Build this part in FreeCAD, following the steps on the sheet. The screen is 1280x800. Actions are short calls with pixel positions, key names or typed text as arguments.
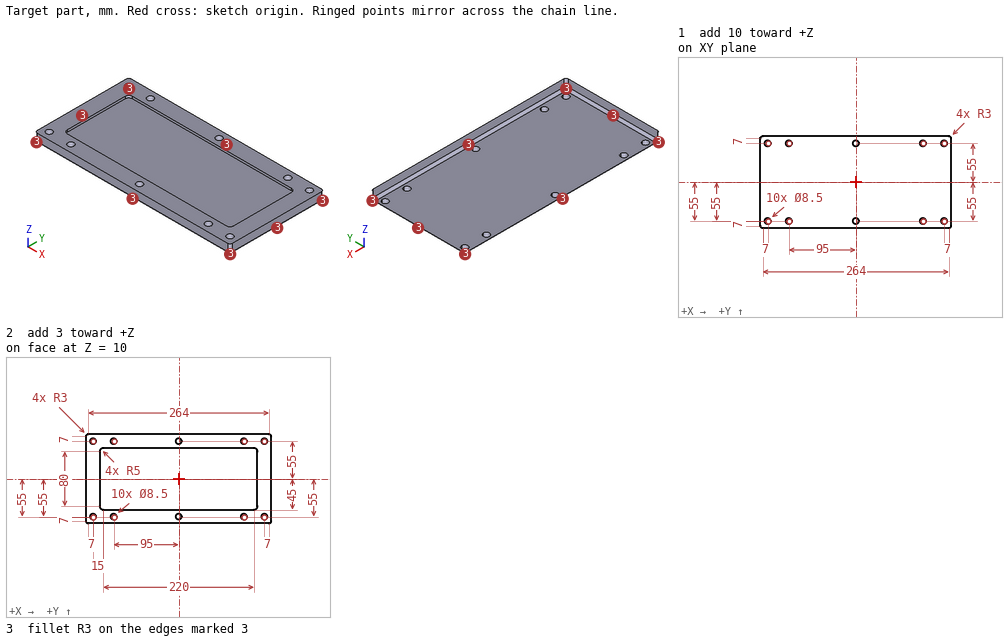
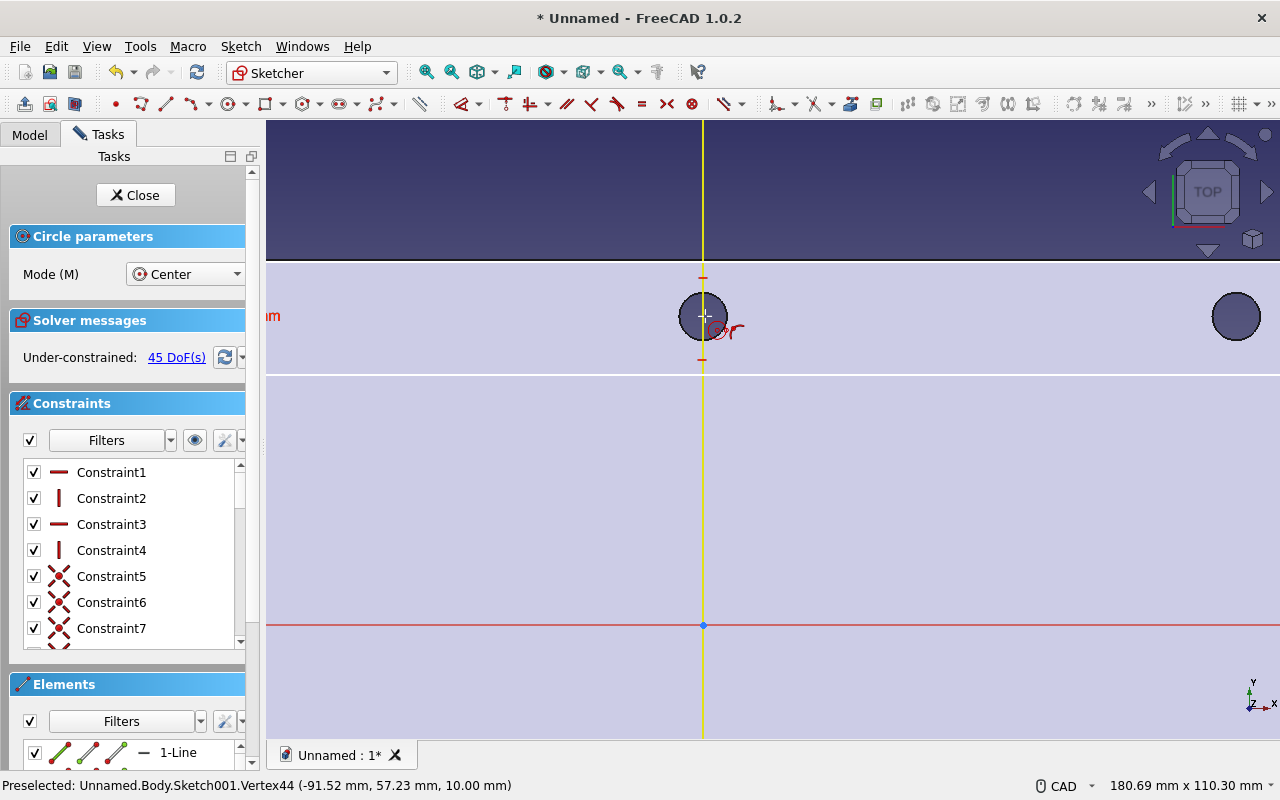
click(703, 317)
move(720, 300)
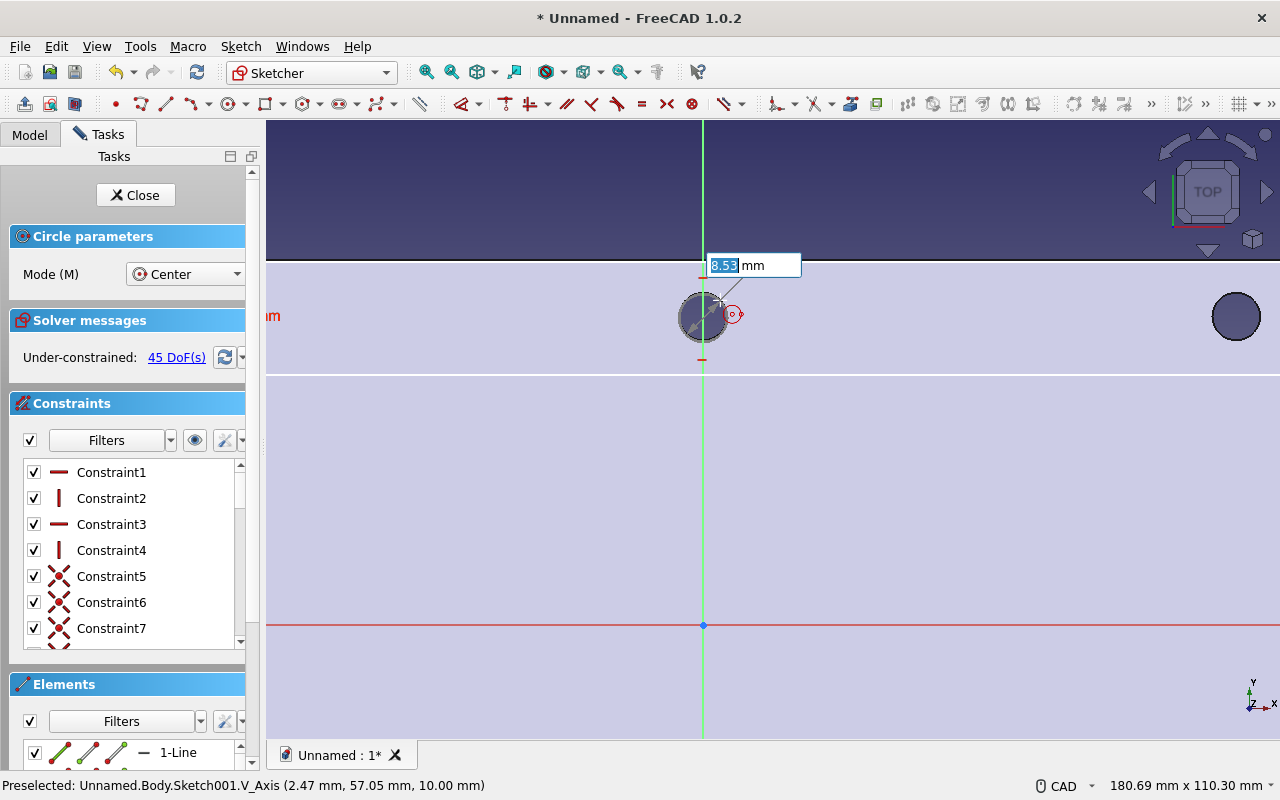
text(8.5)
key(Return)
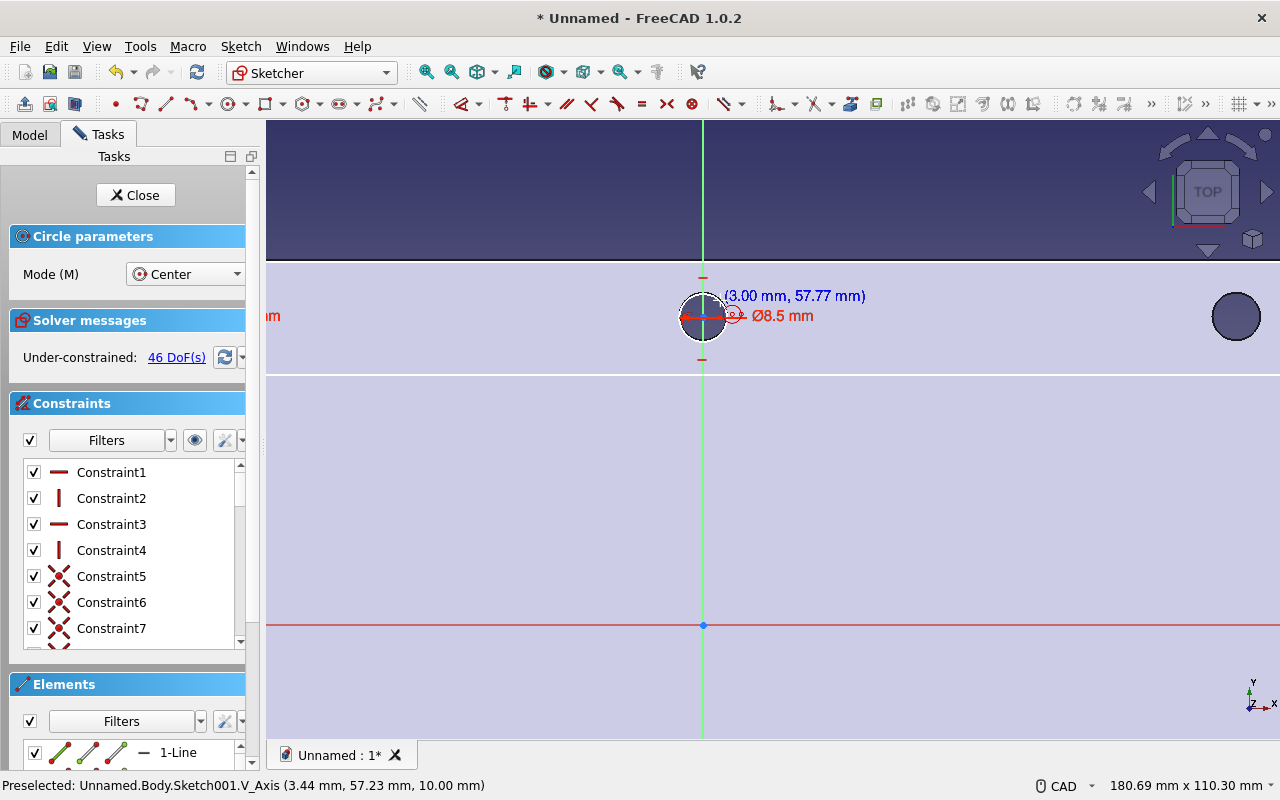
scroll(705, 316, down, 5)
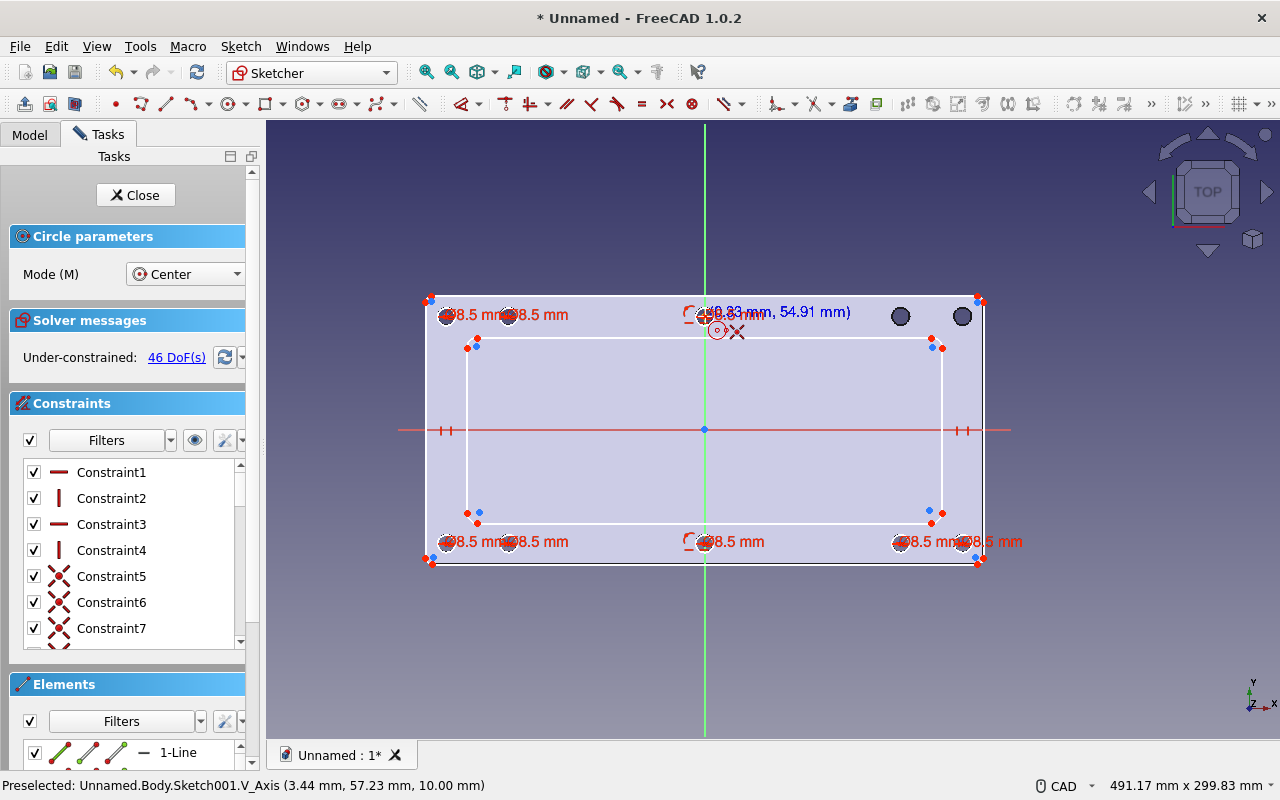
scroll(901, 316, up, 5)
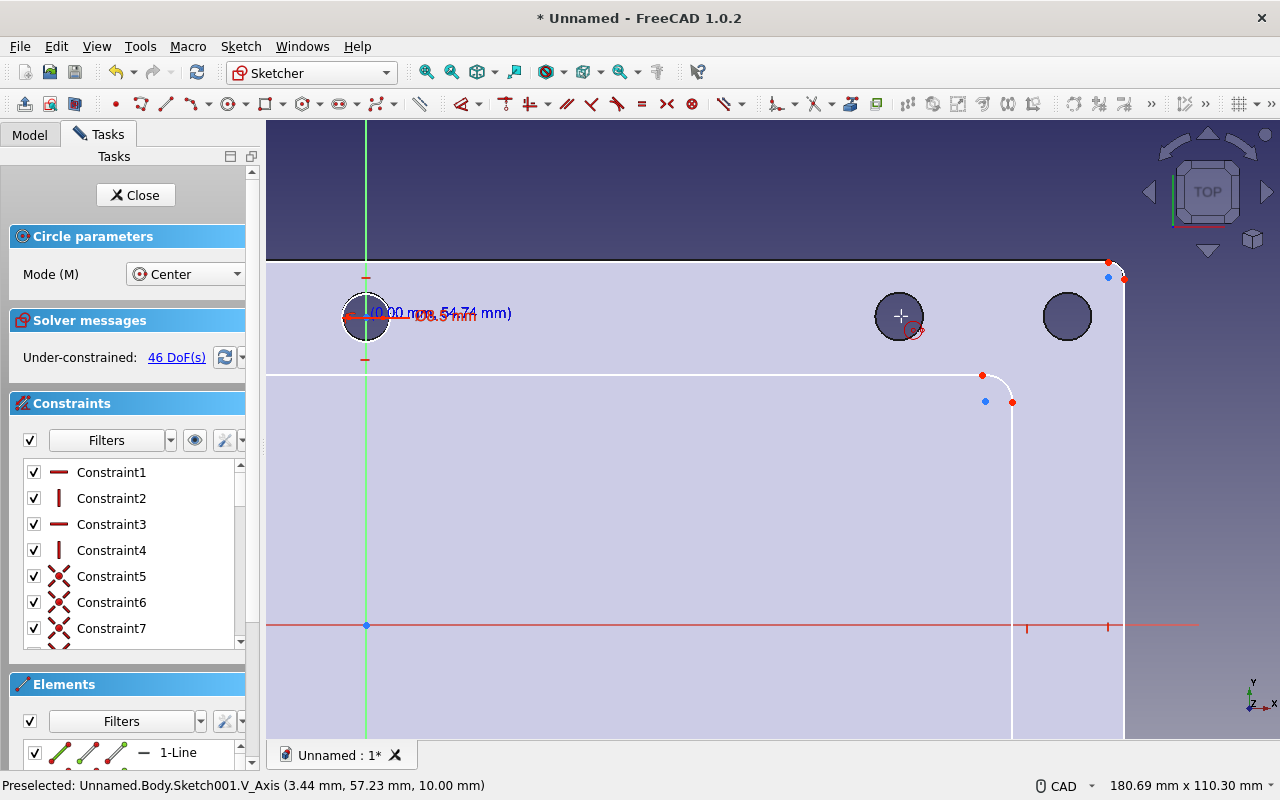
click(899, 317)
move(916, 300)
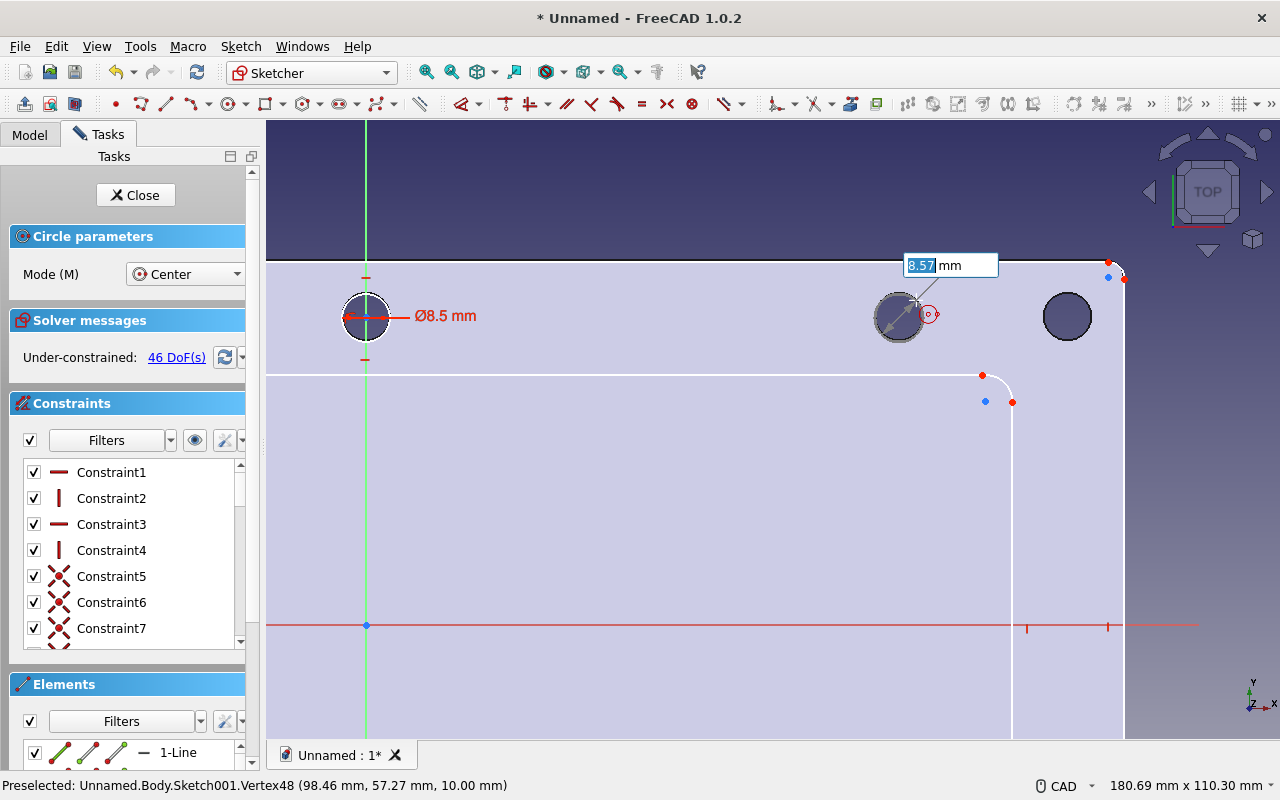
text(8.5)
key(Return)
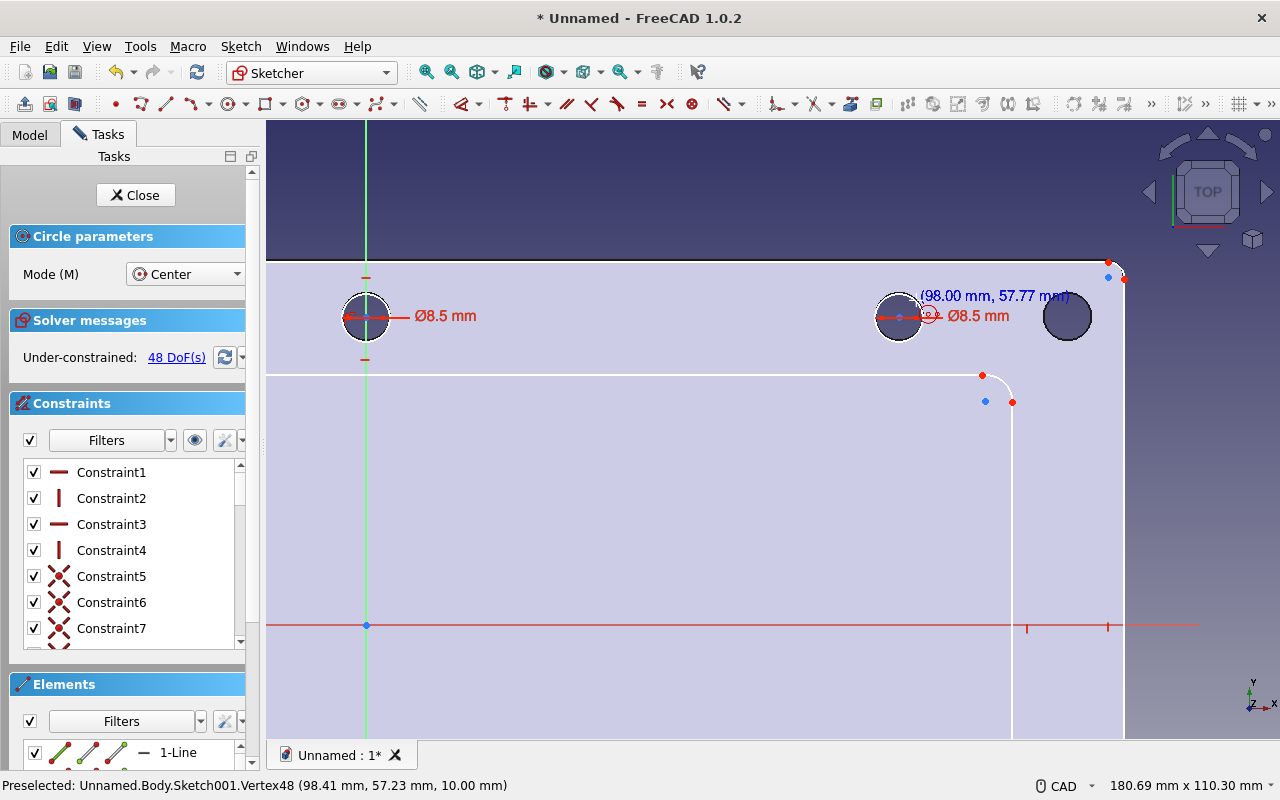
click(1068, 317)
move(1084, 300)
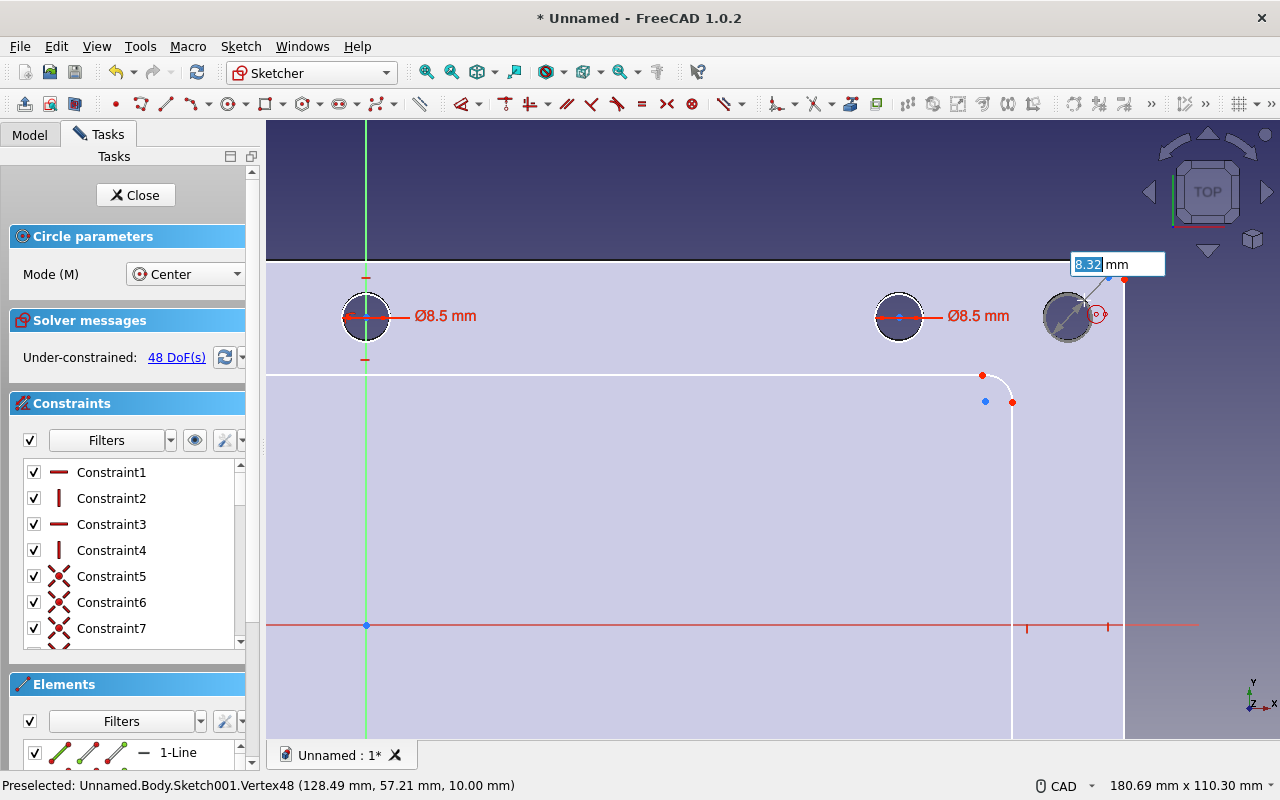
text(8.5)
key(Return)
key(Escape)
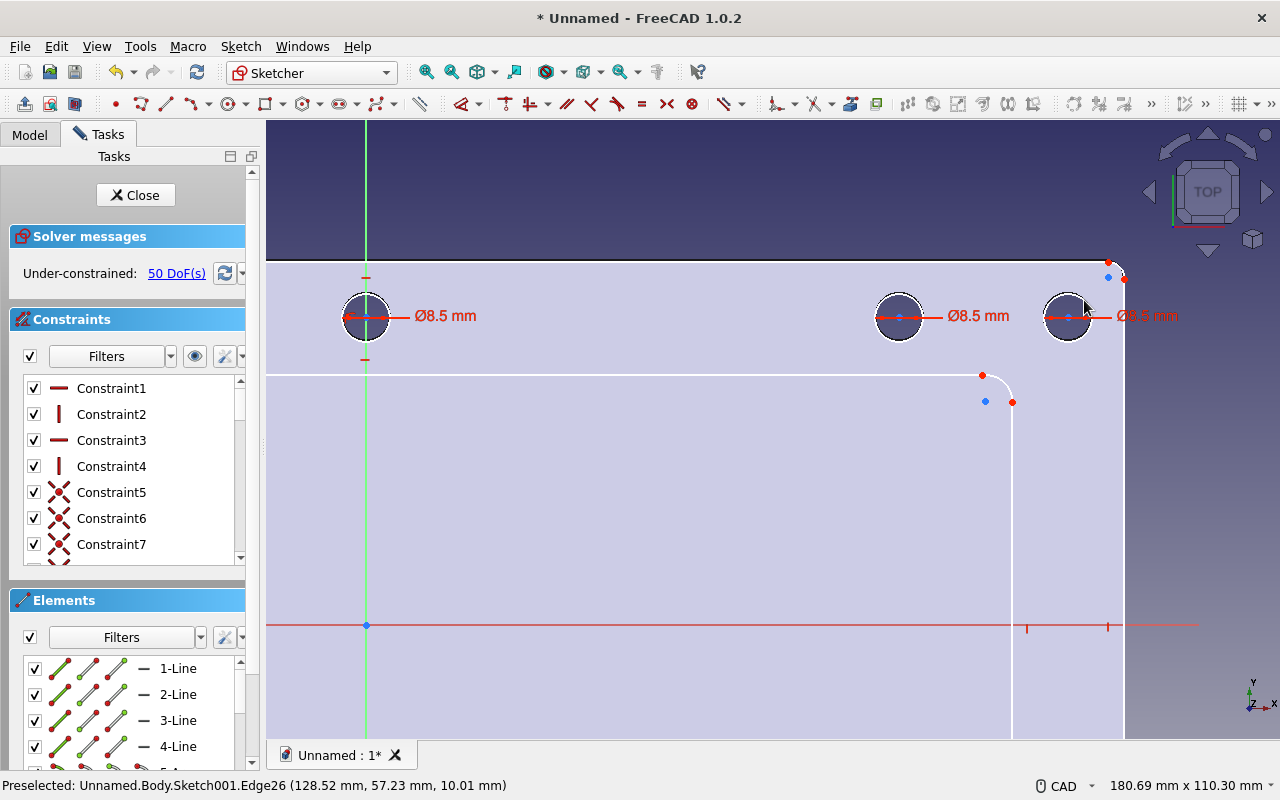
click(663, 262)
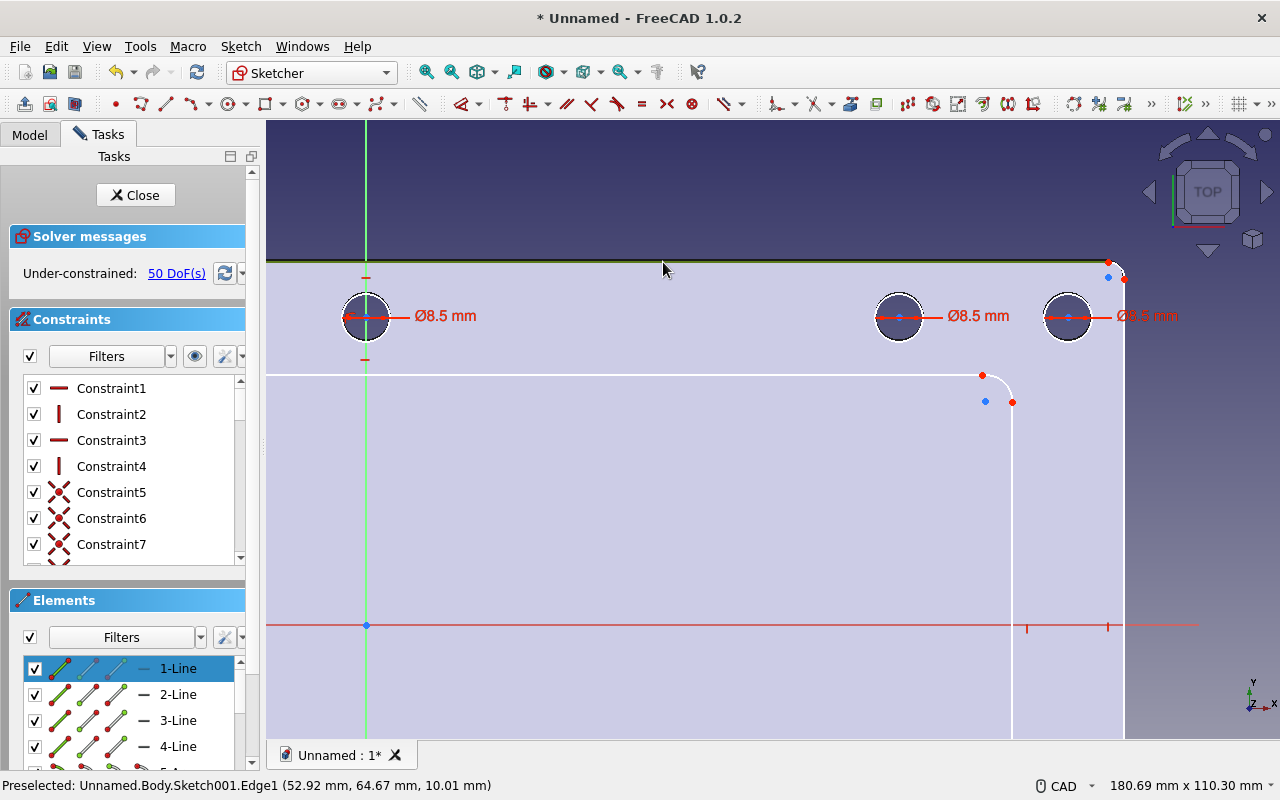
scroll(901, 316, down, 5)